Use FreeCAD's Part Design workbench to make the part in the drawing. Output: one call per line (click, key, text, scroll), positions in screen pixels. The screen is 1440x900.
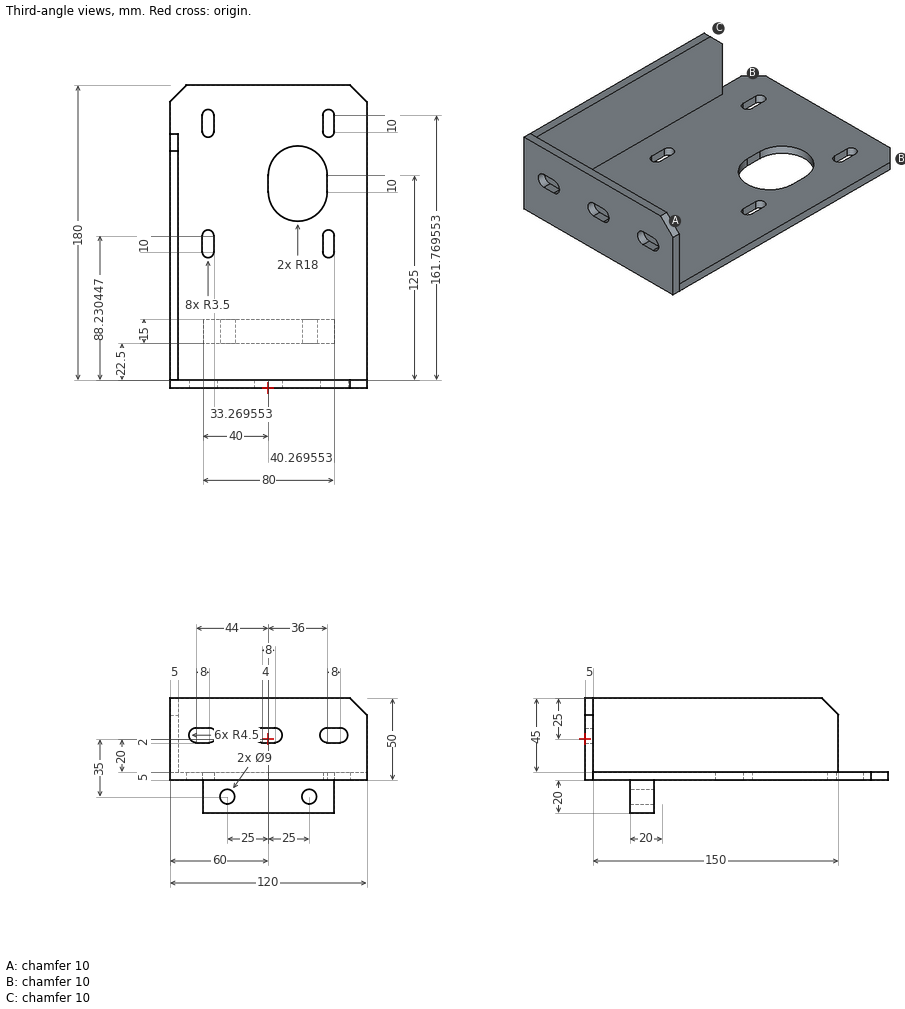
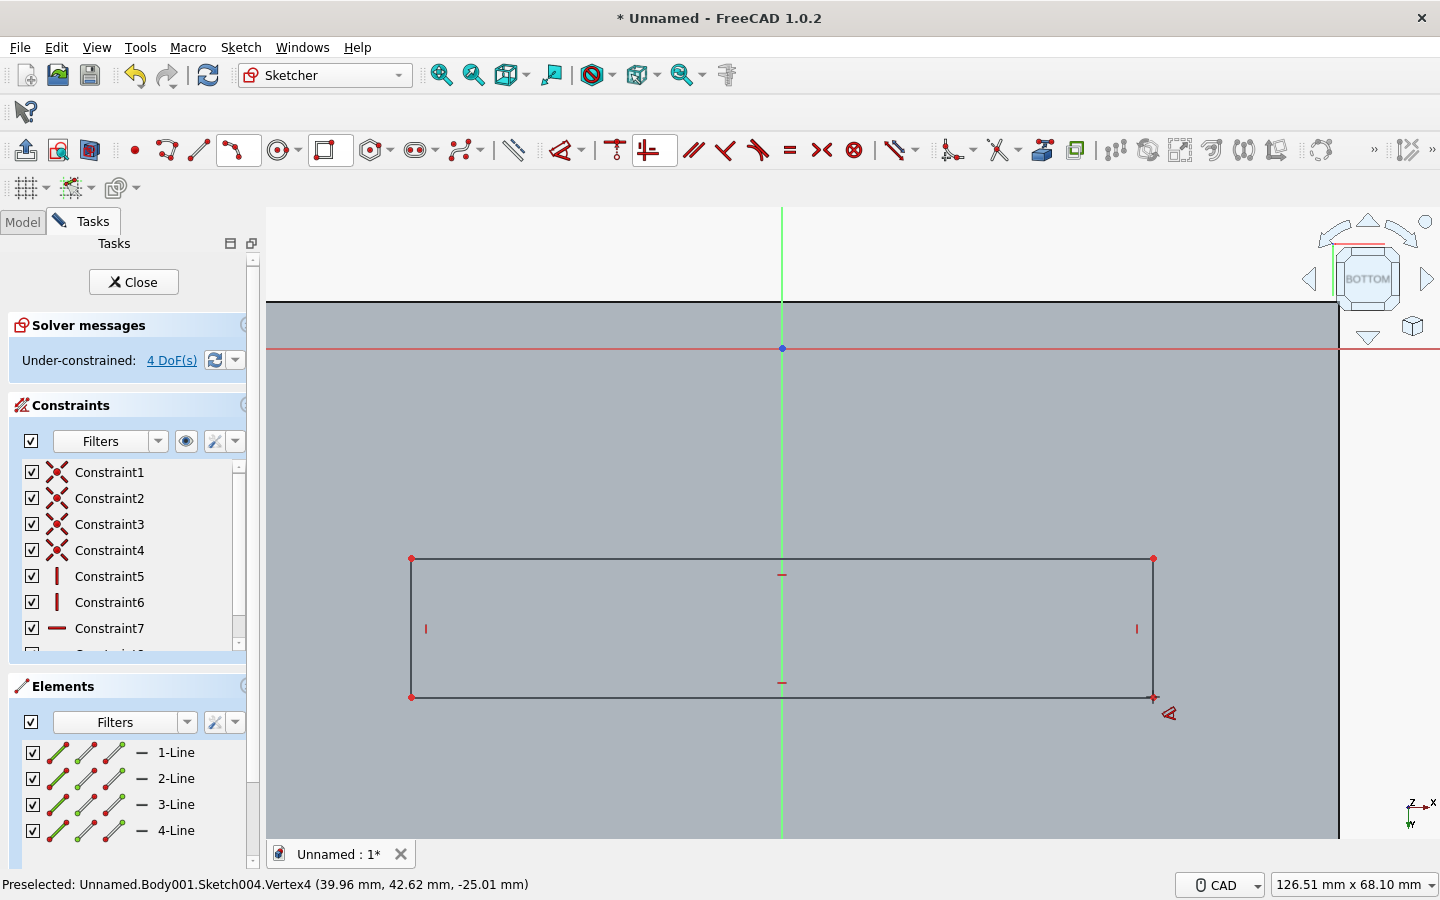
click(411, 601)
click(377, 628)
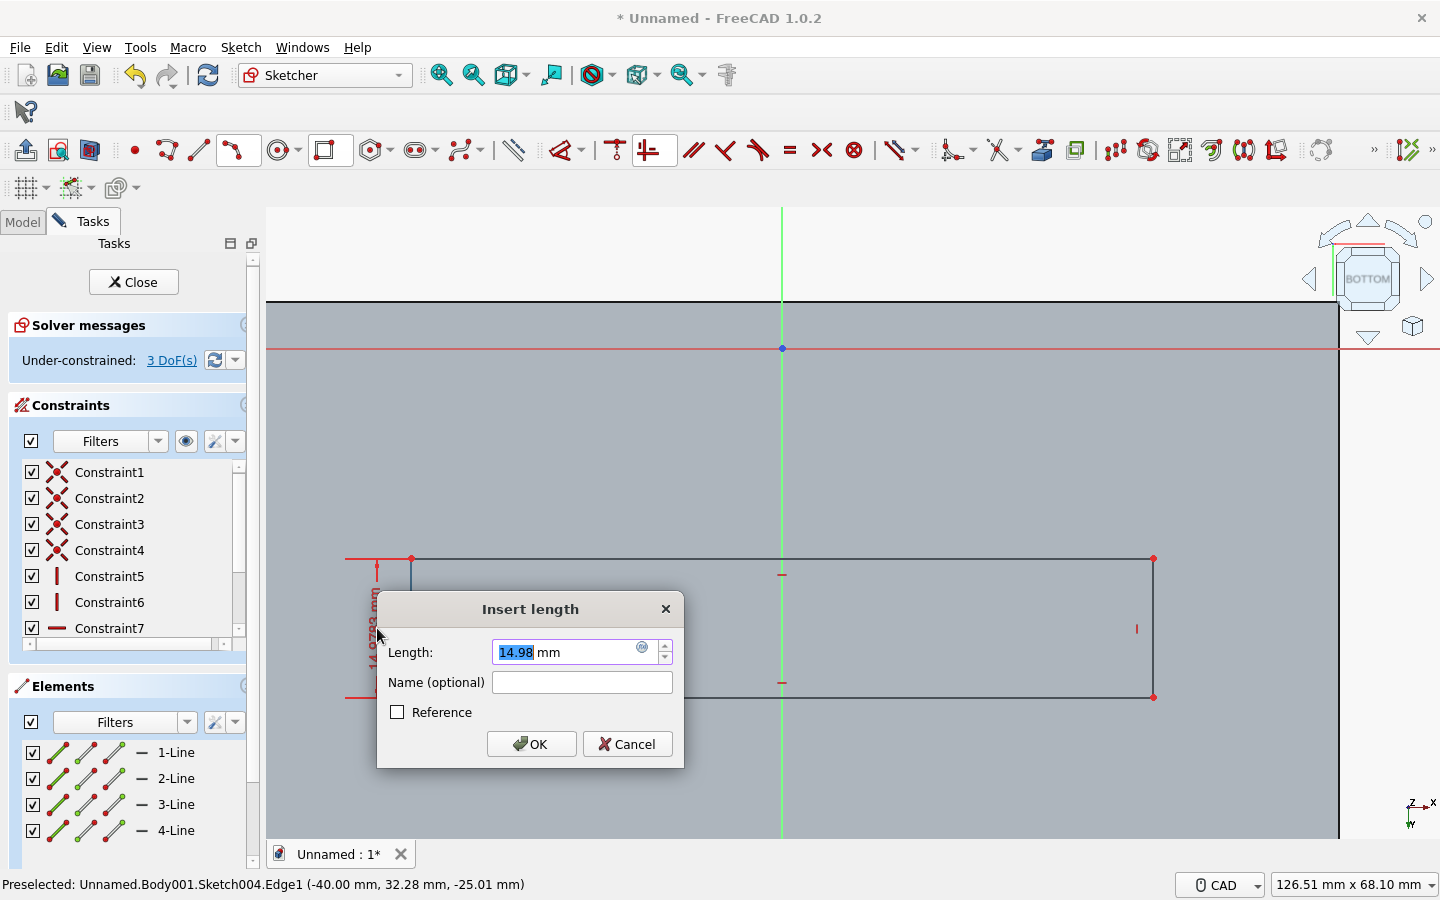
text(15)
key(Return)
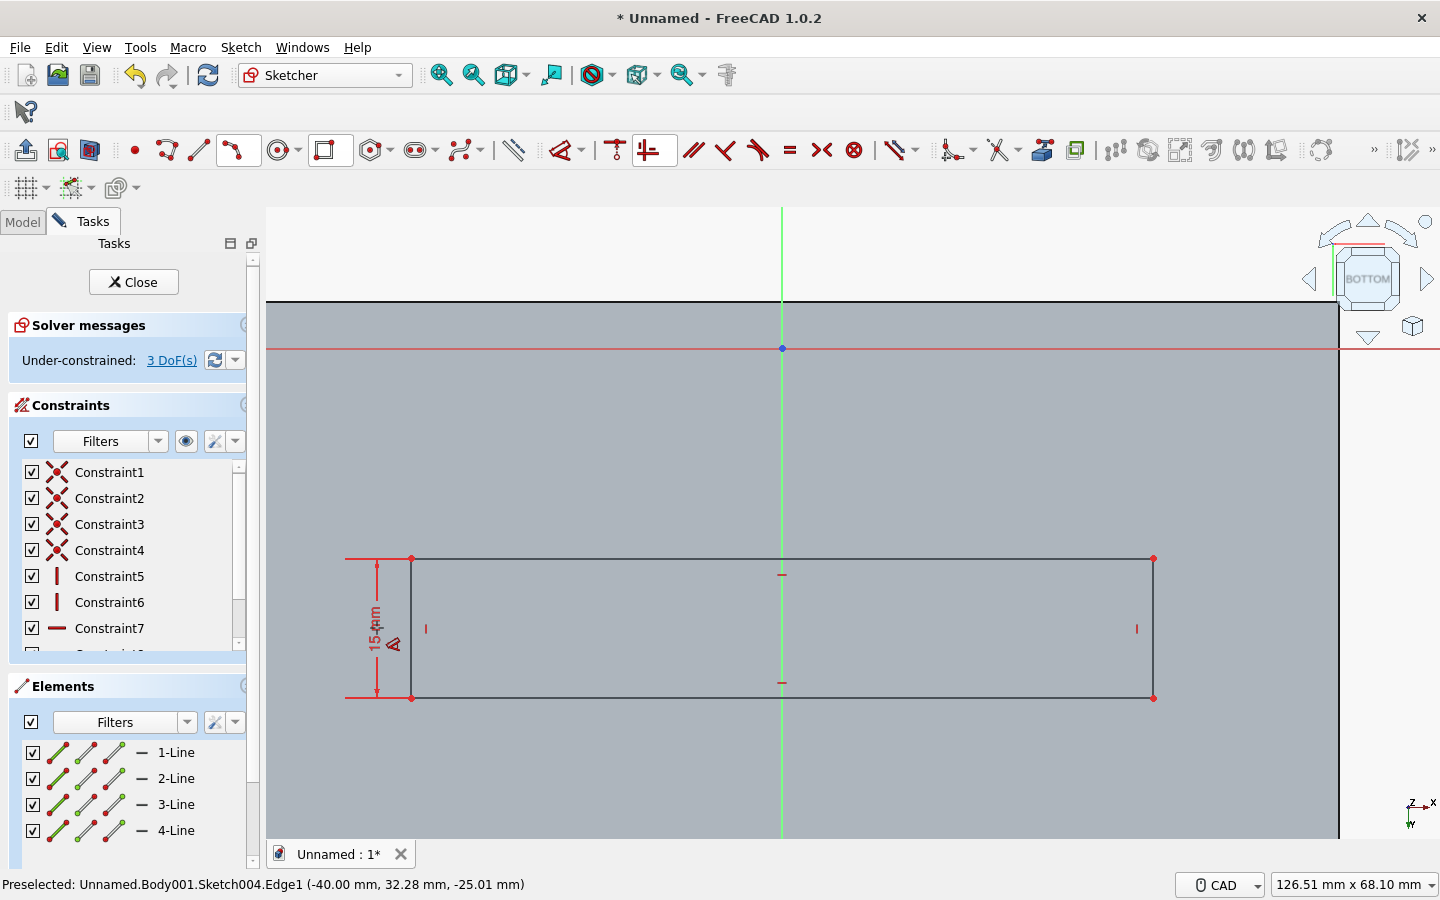
click(634, 698)
click(611, 732)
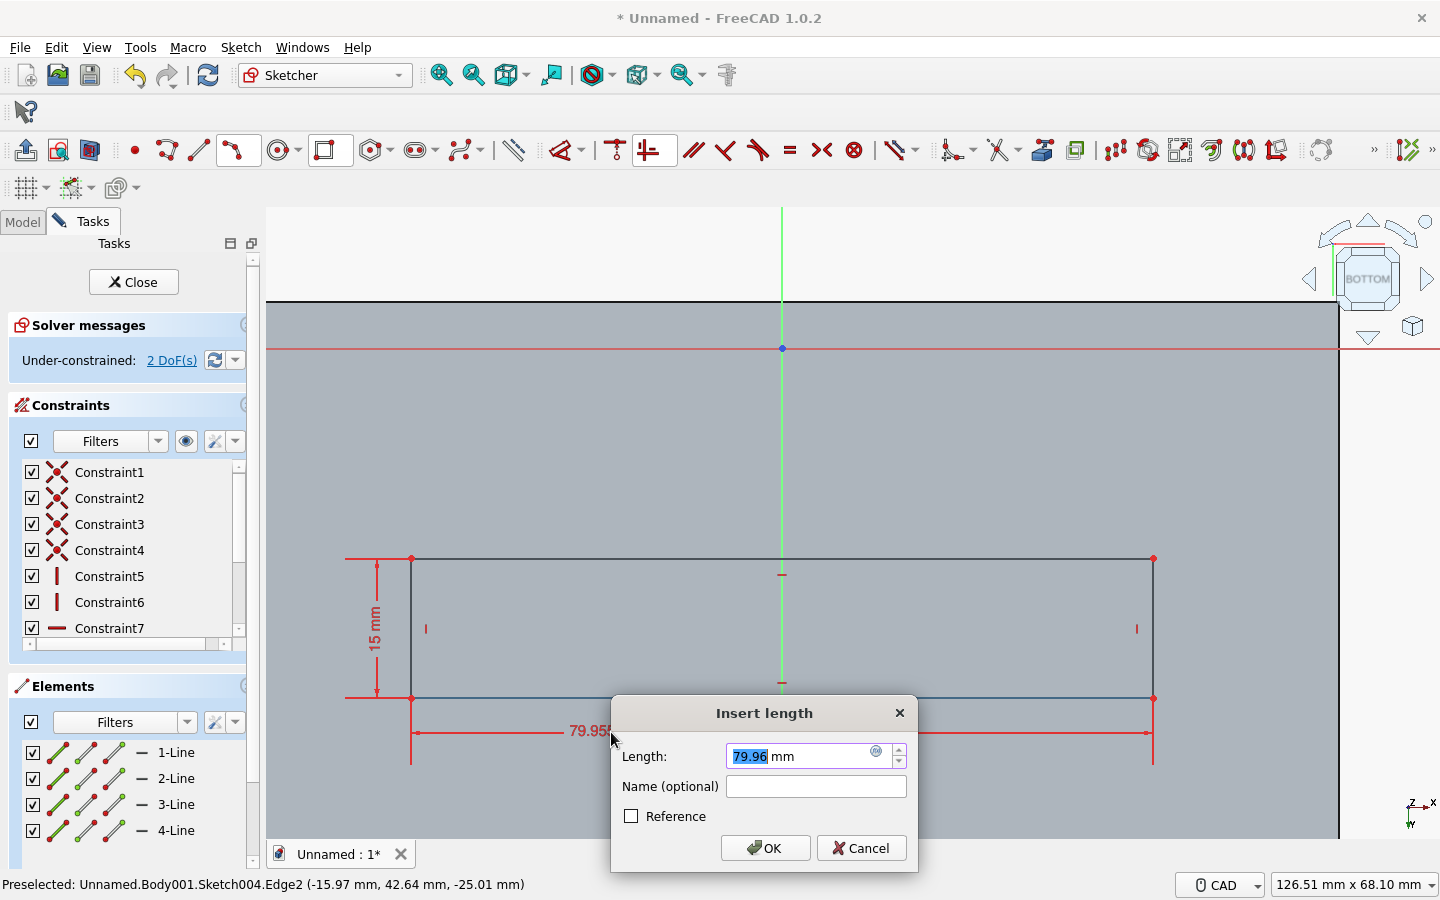
text(80)
key(Return)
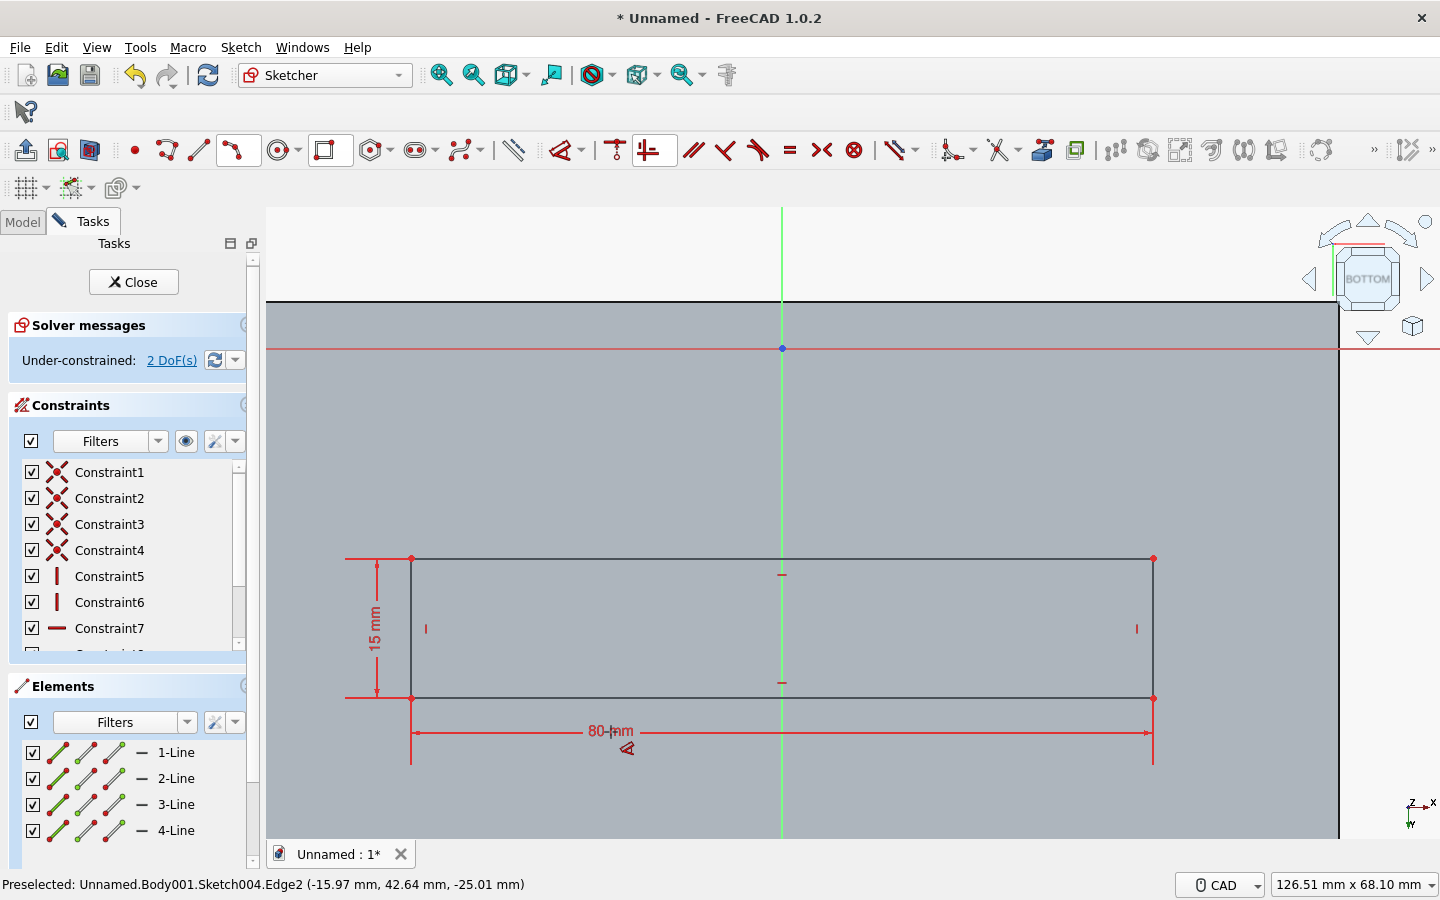
click(411, 559)
click(597, 315)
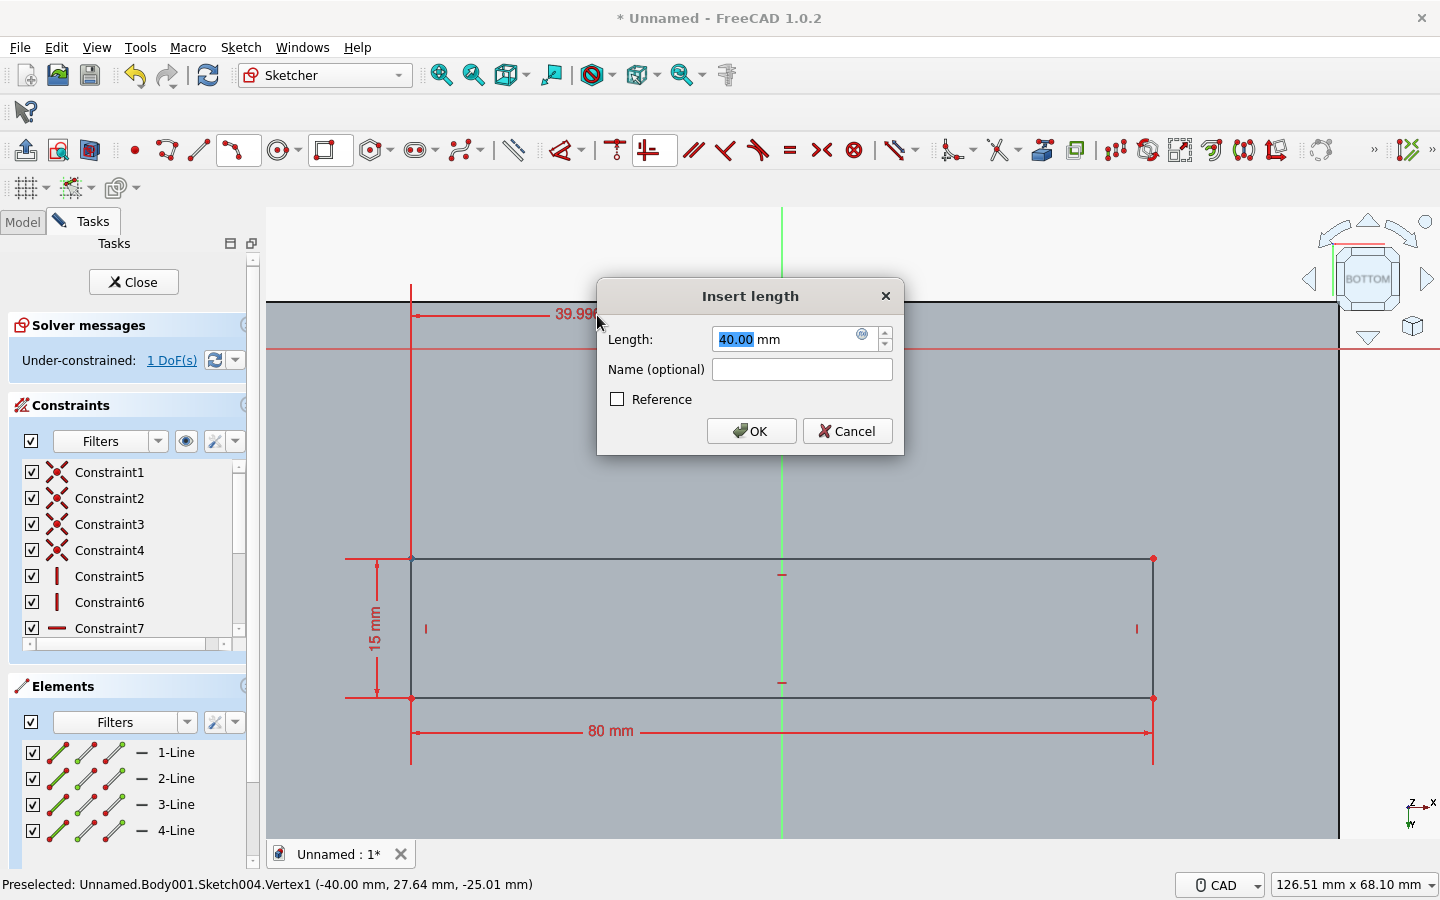
text(40)
key(Return)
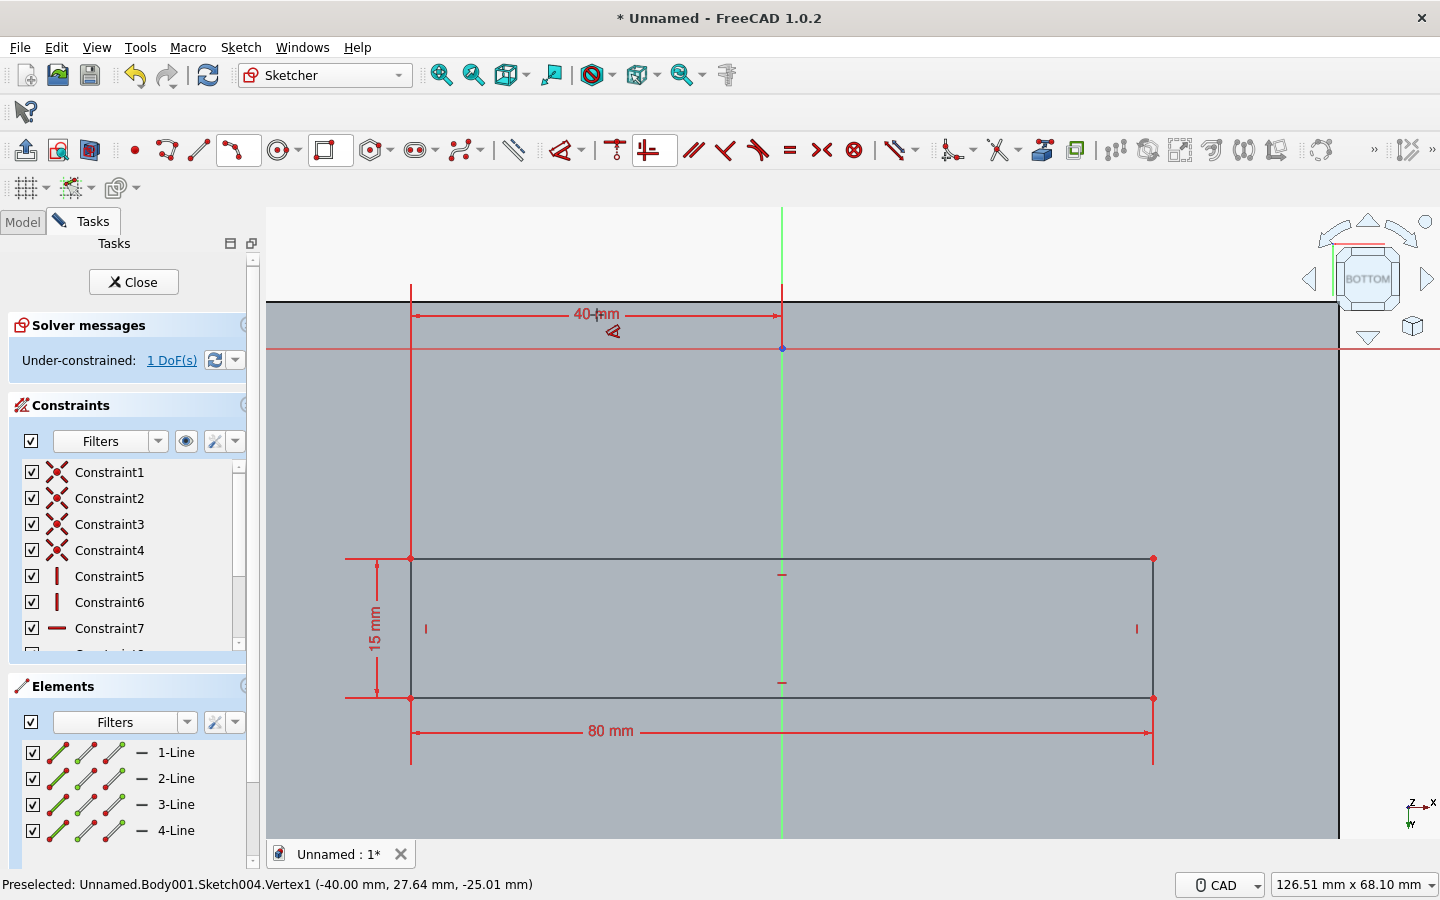
click(411, 559)
click(377, 454)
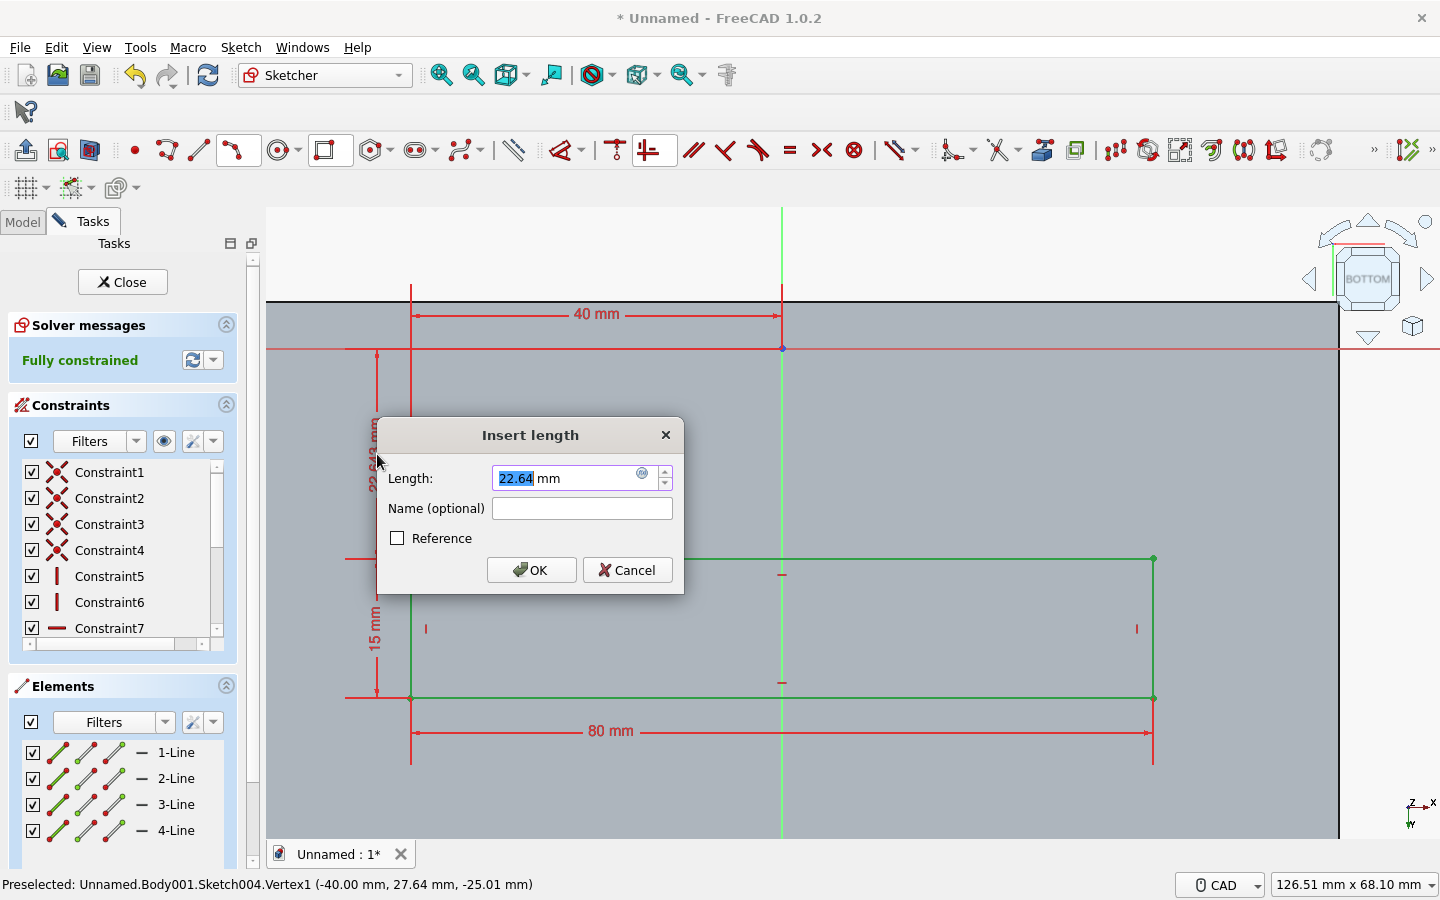
text(22.5)
key(Return)
key(Escape)